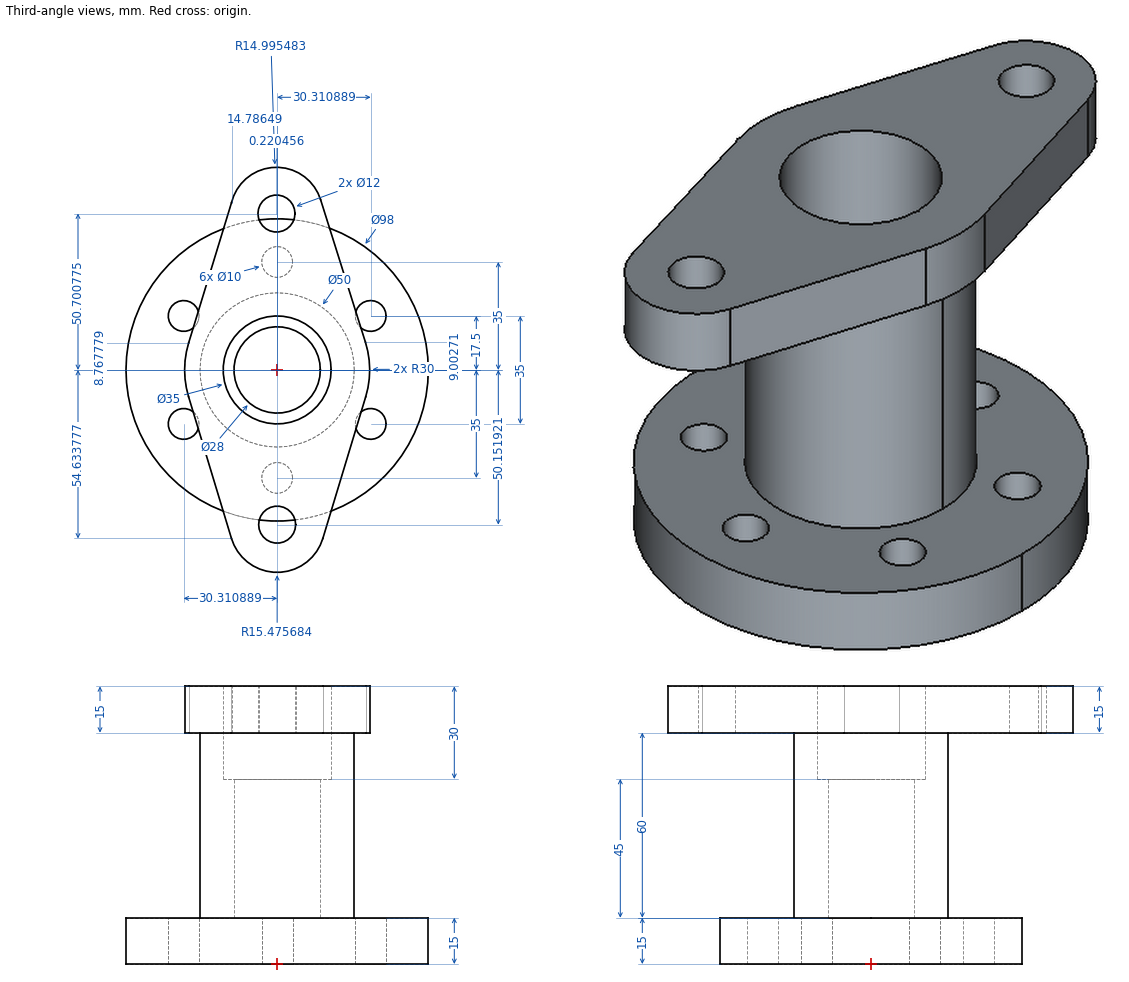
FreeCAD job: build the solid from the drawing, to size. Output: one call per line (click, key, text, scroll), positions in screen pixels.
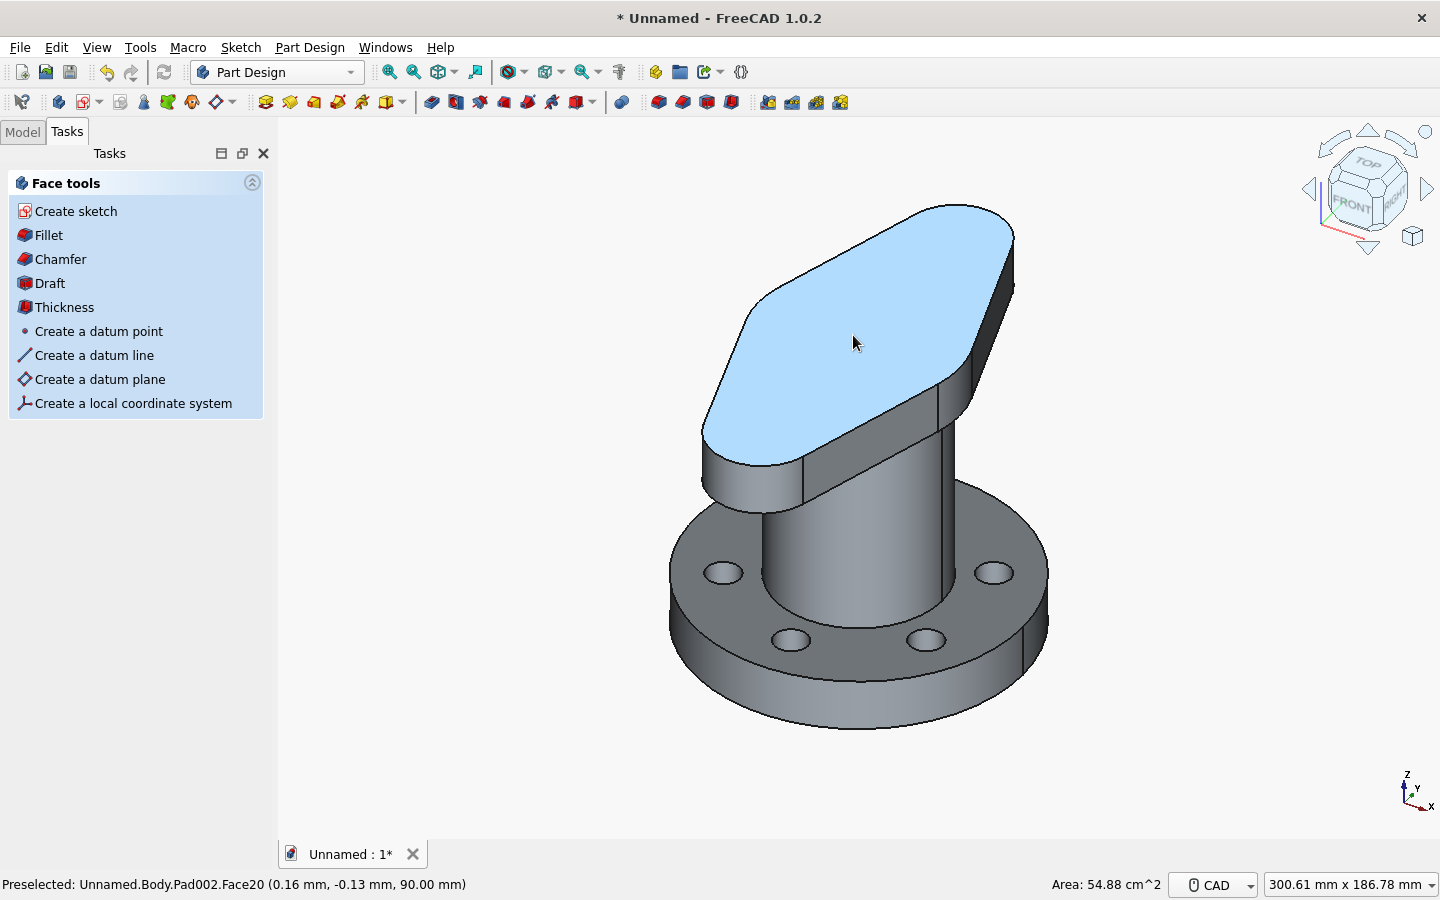
click(84, 102)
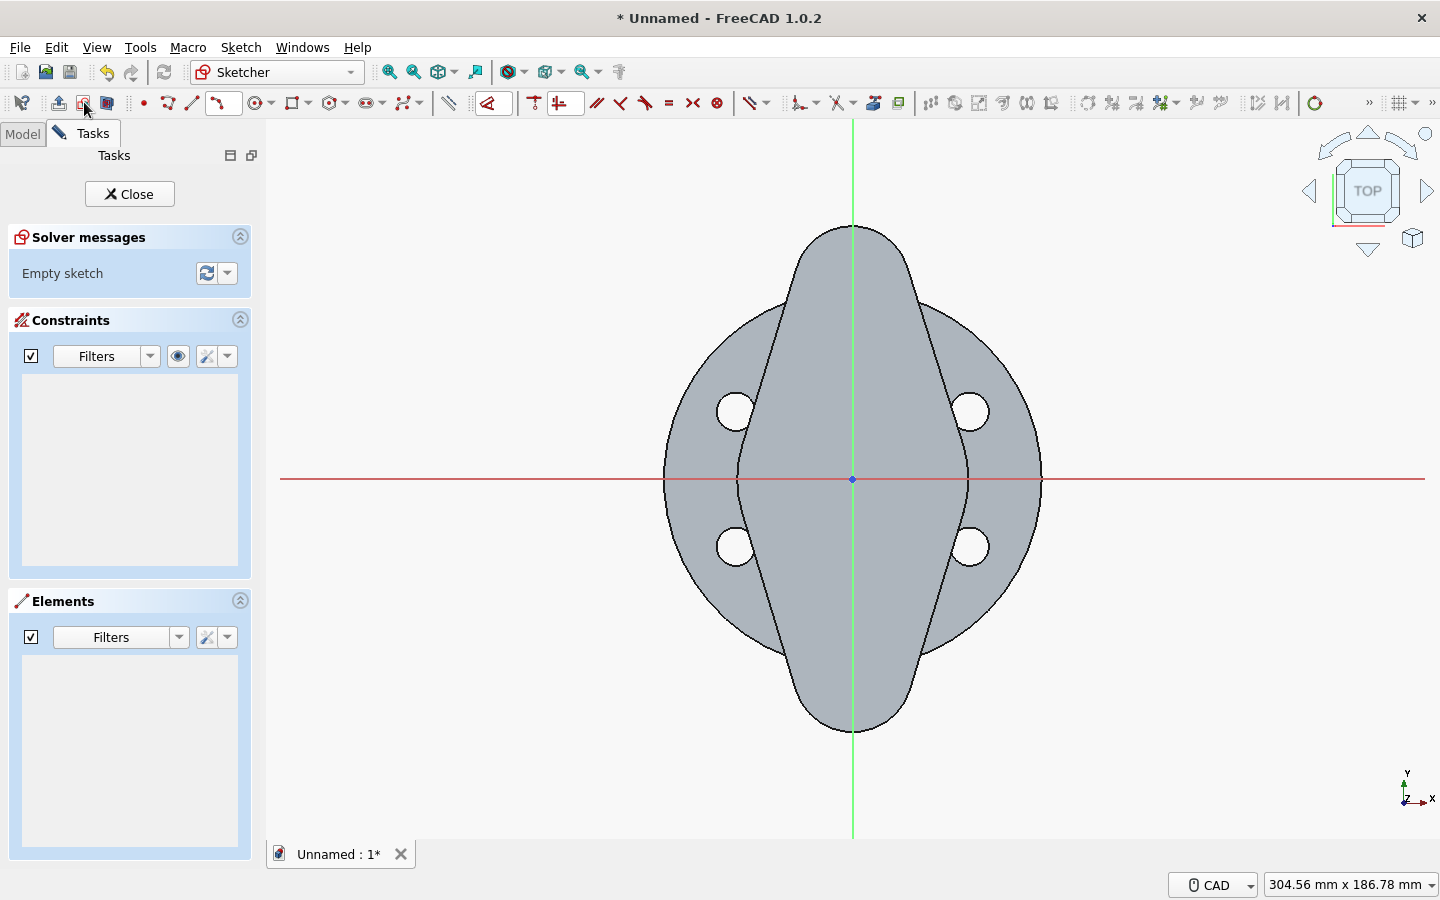
key(g)
key(c)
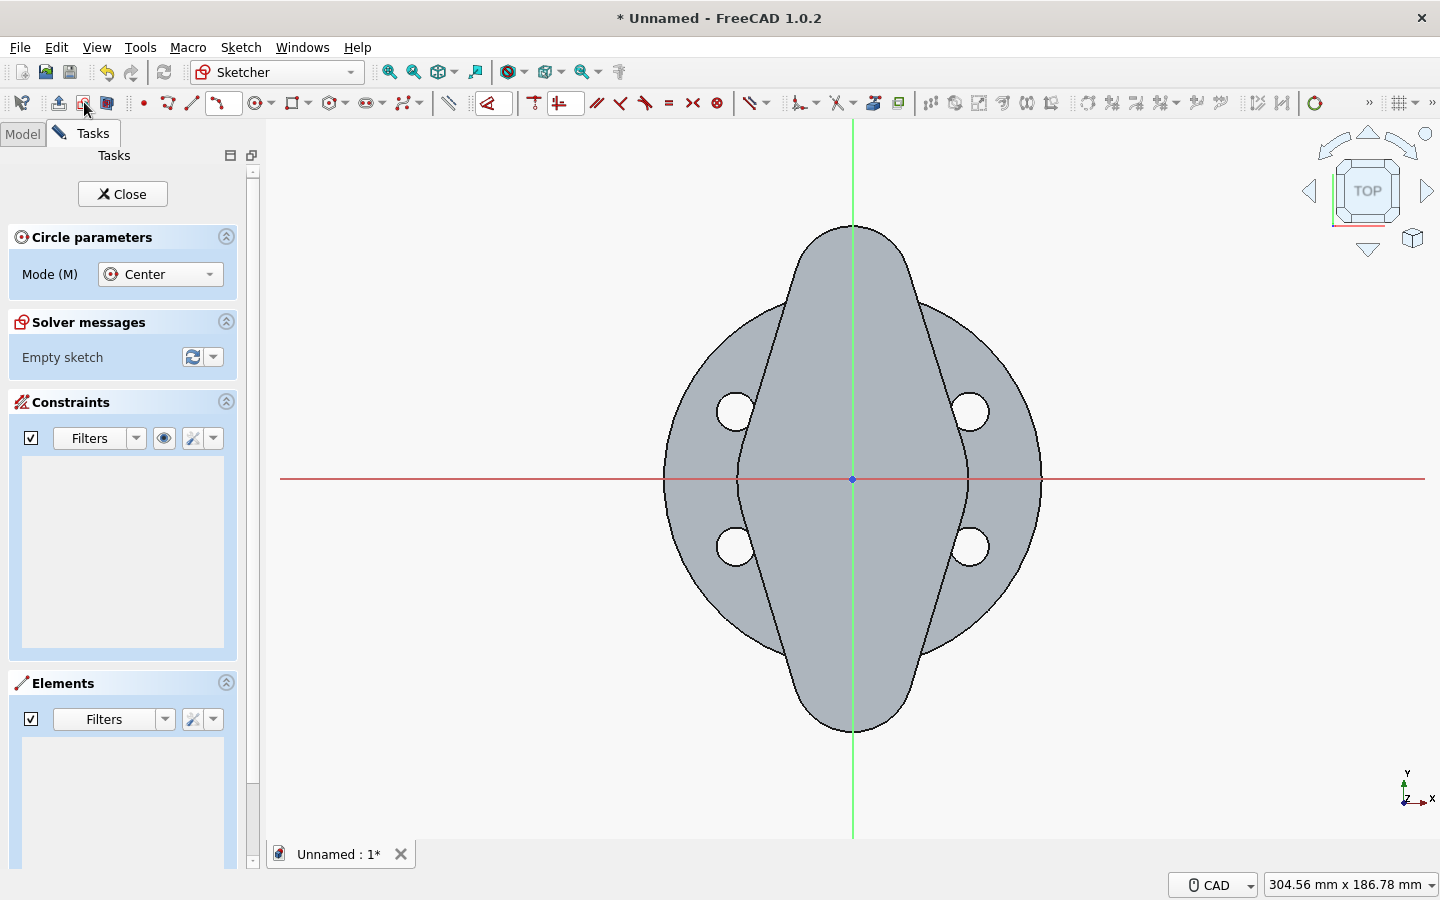
scroll(852, 284, up, 15)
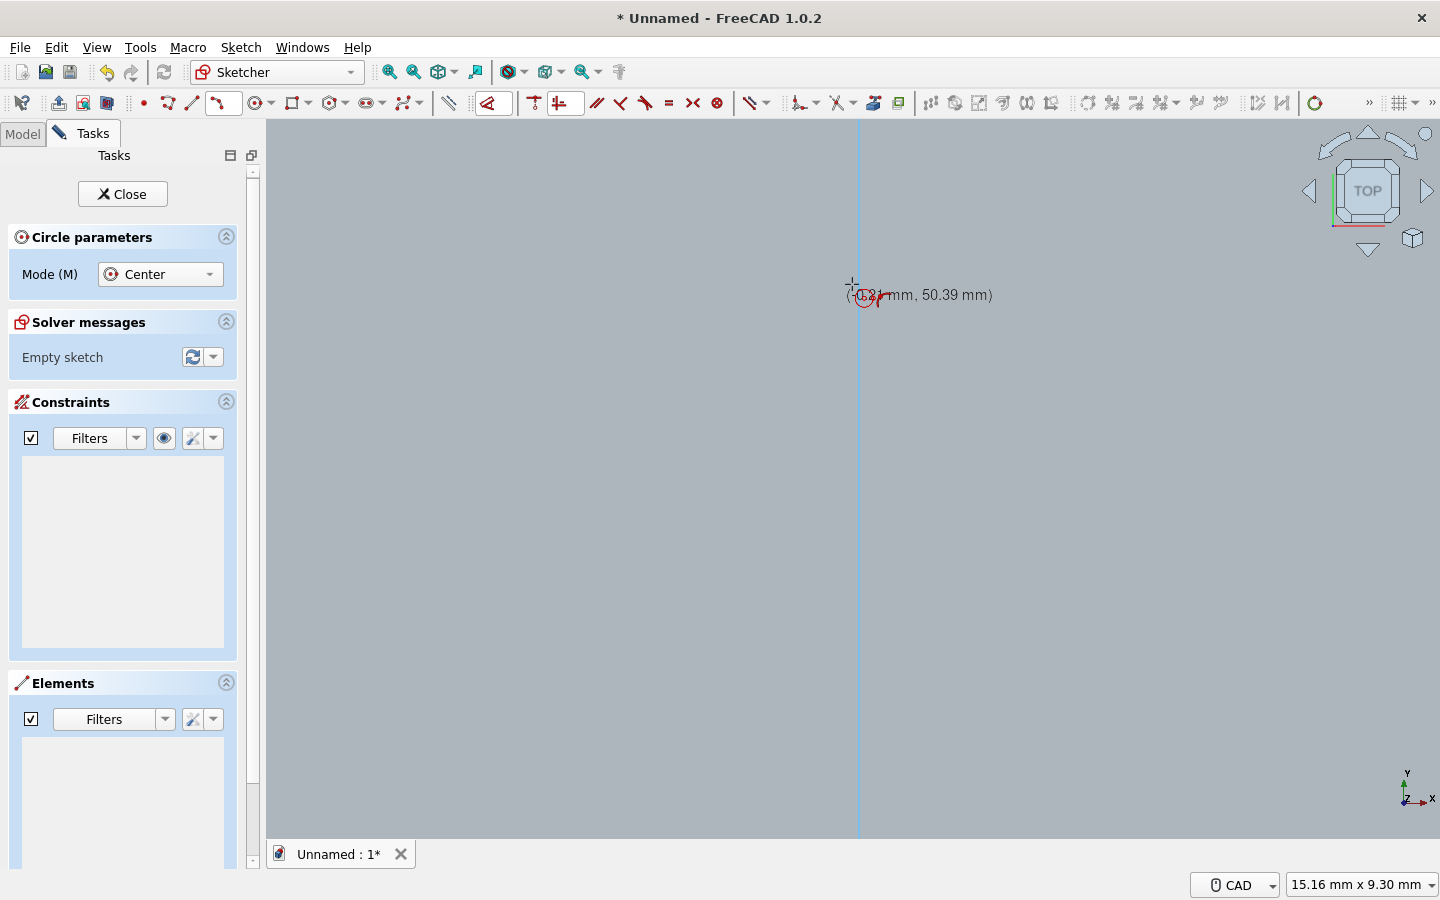
click(842, 275)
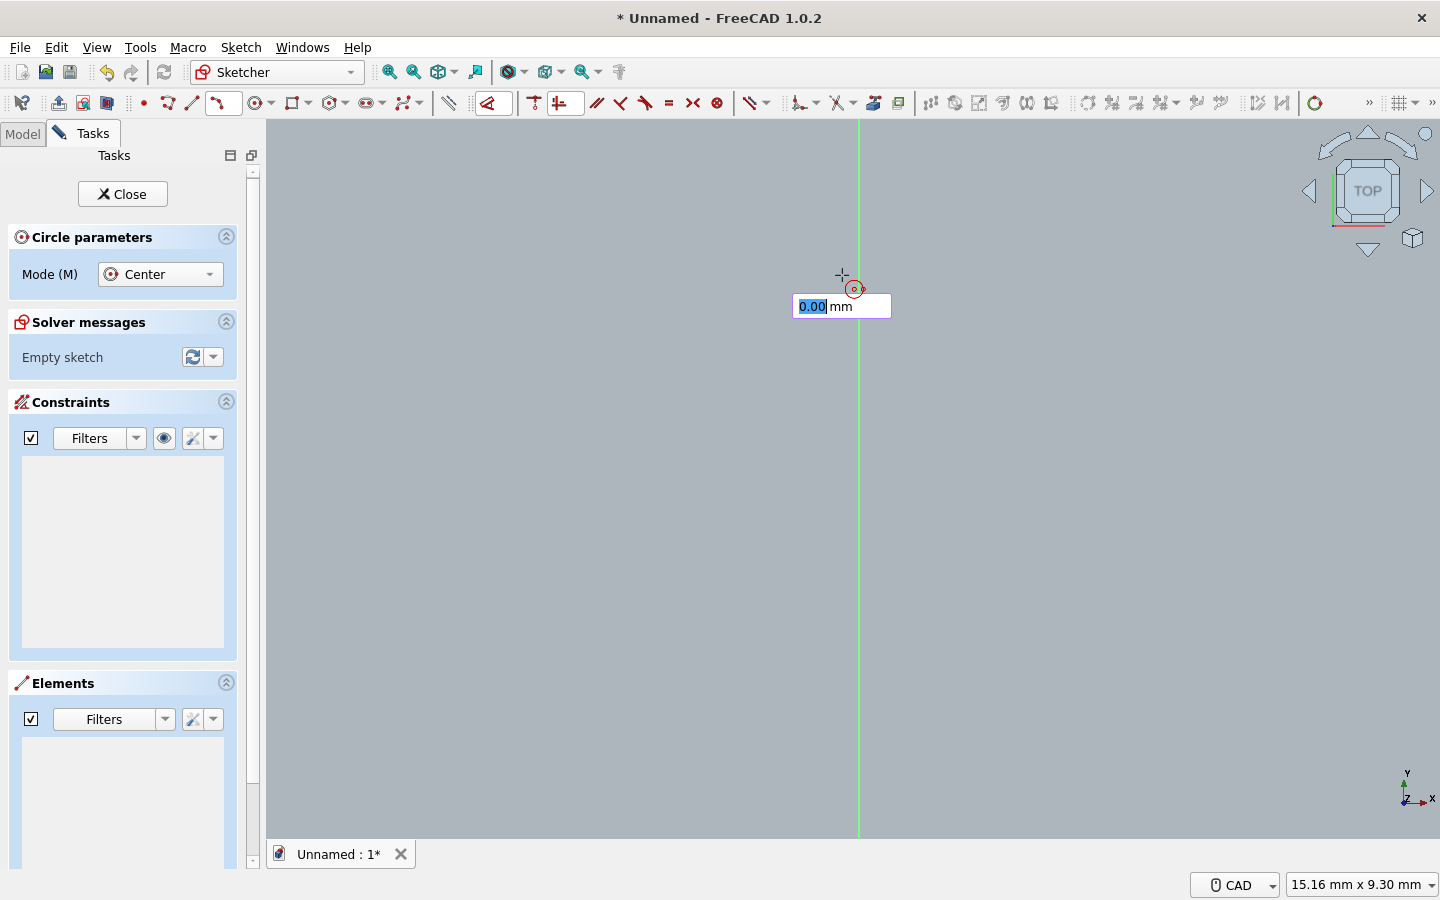
scroll(781, 285, down, 15)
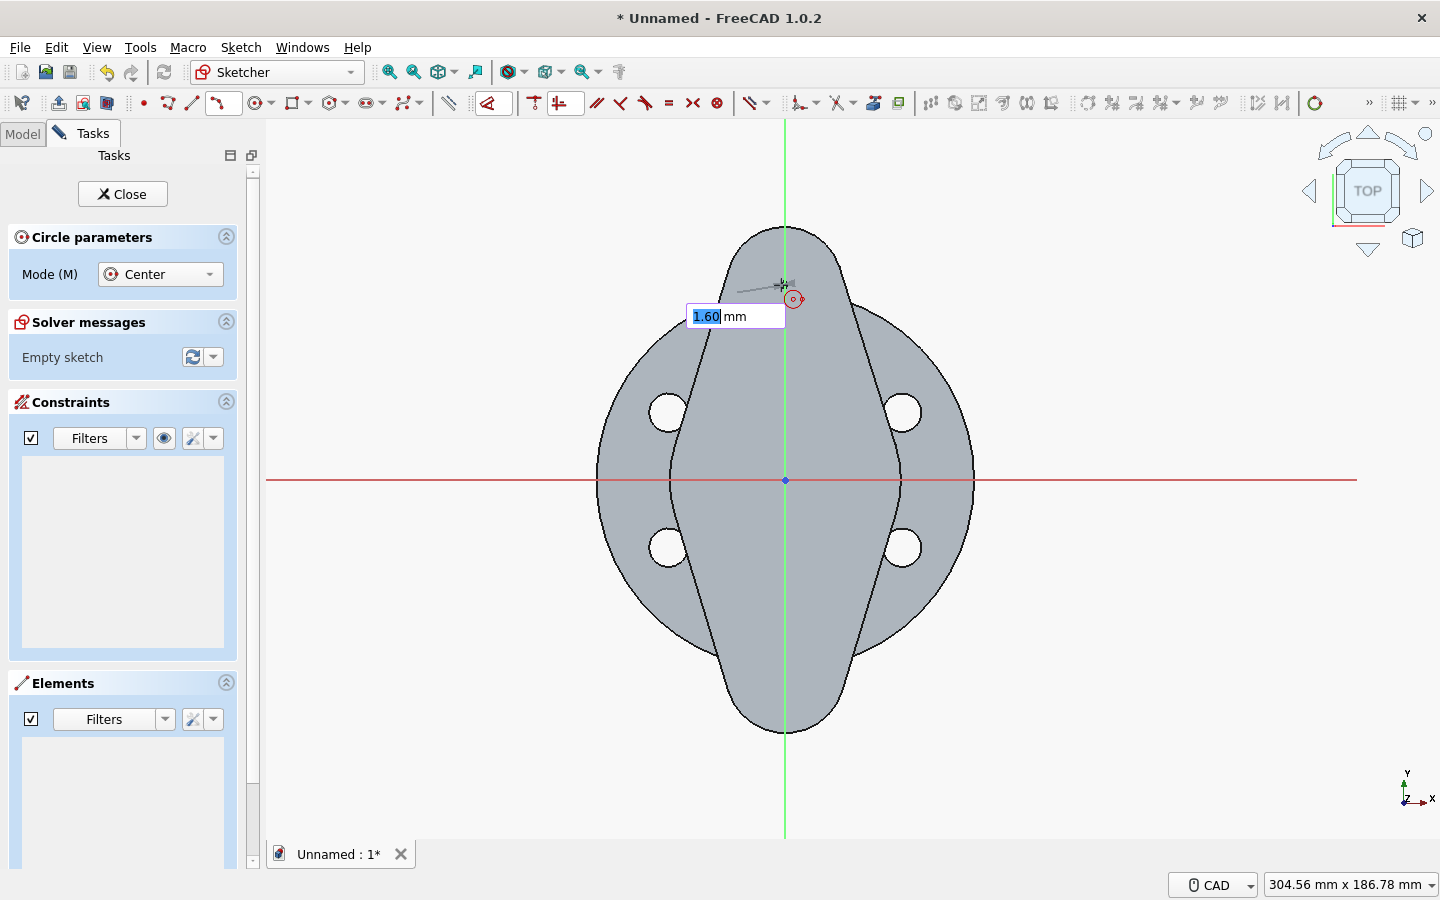
click(801, 268)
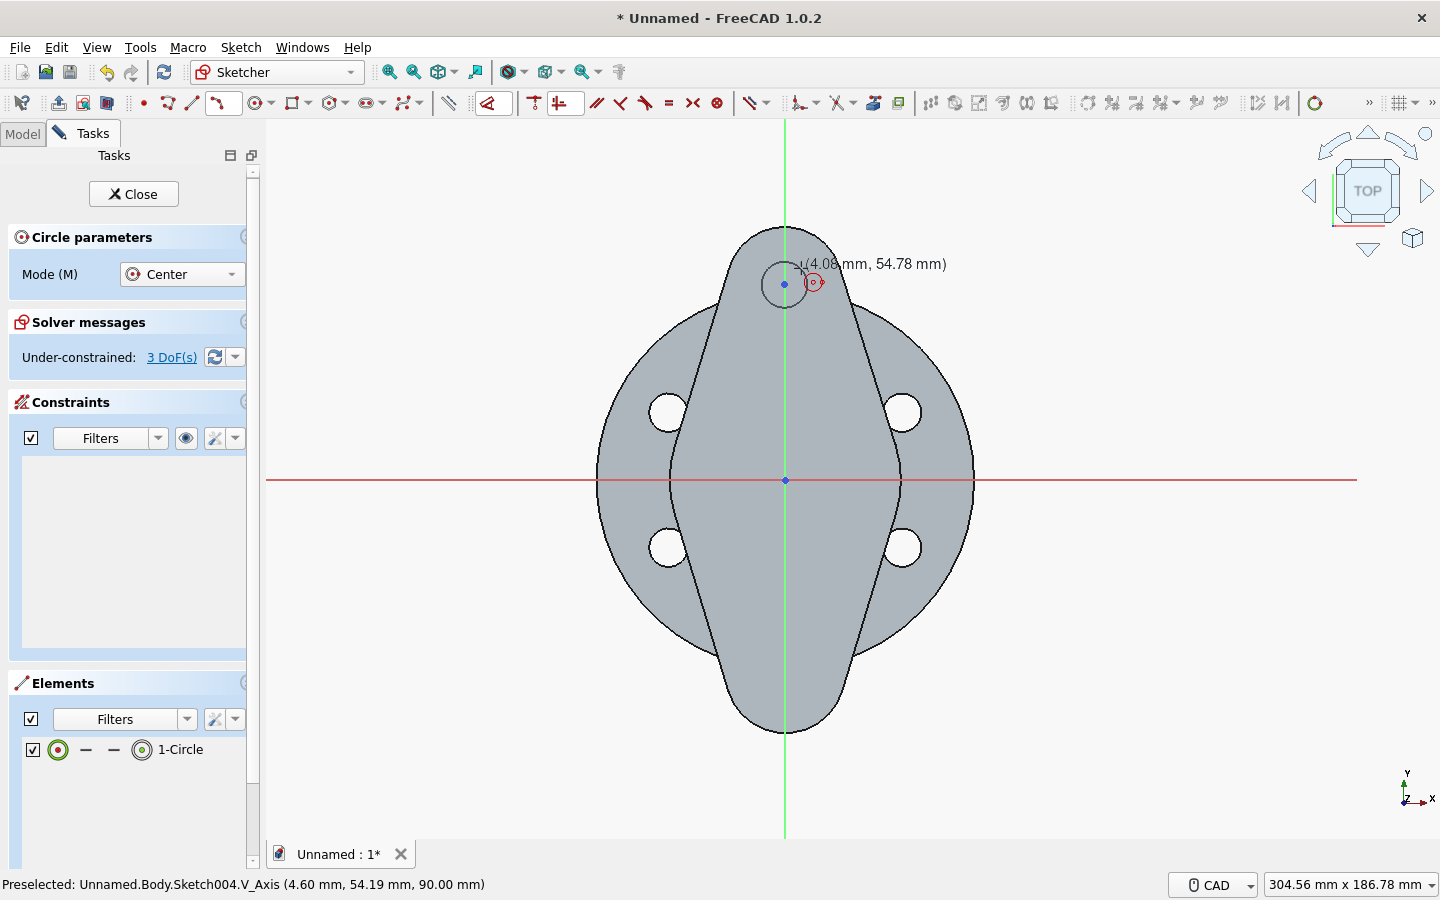
click(785, 673)
click(802, 657)
key(Escape)